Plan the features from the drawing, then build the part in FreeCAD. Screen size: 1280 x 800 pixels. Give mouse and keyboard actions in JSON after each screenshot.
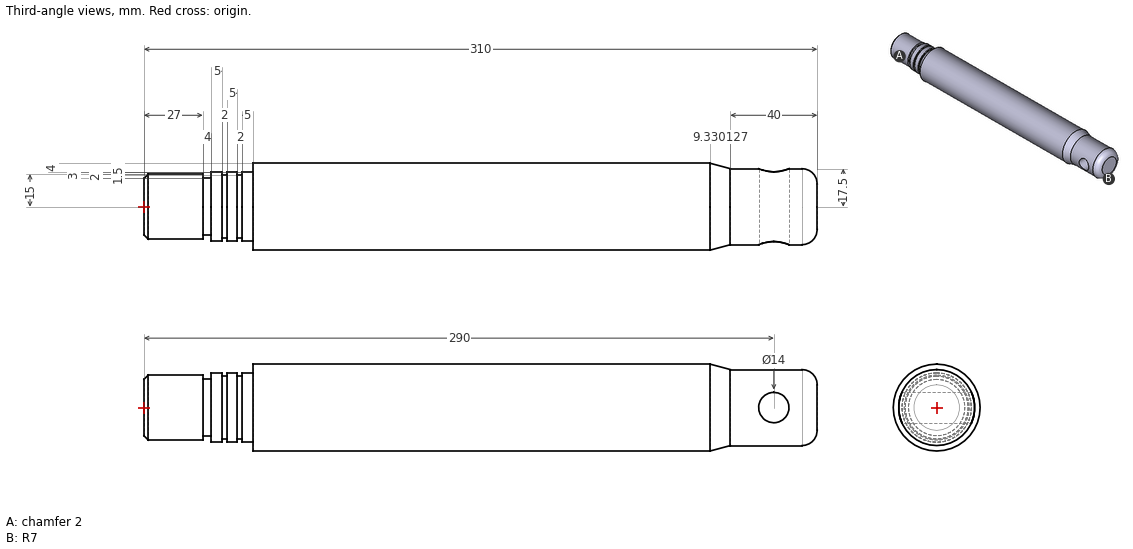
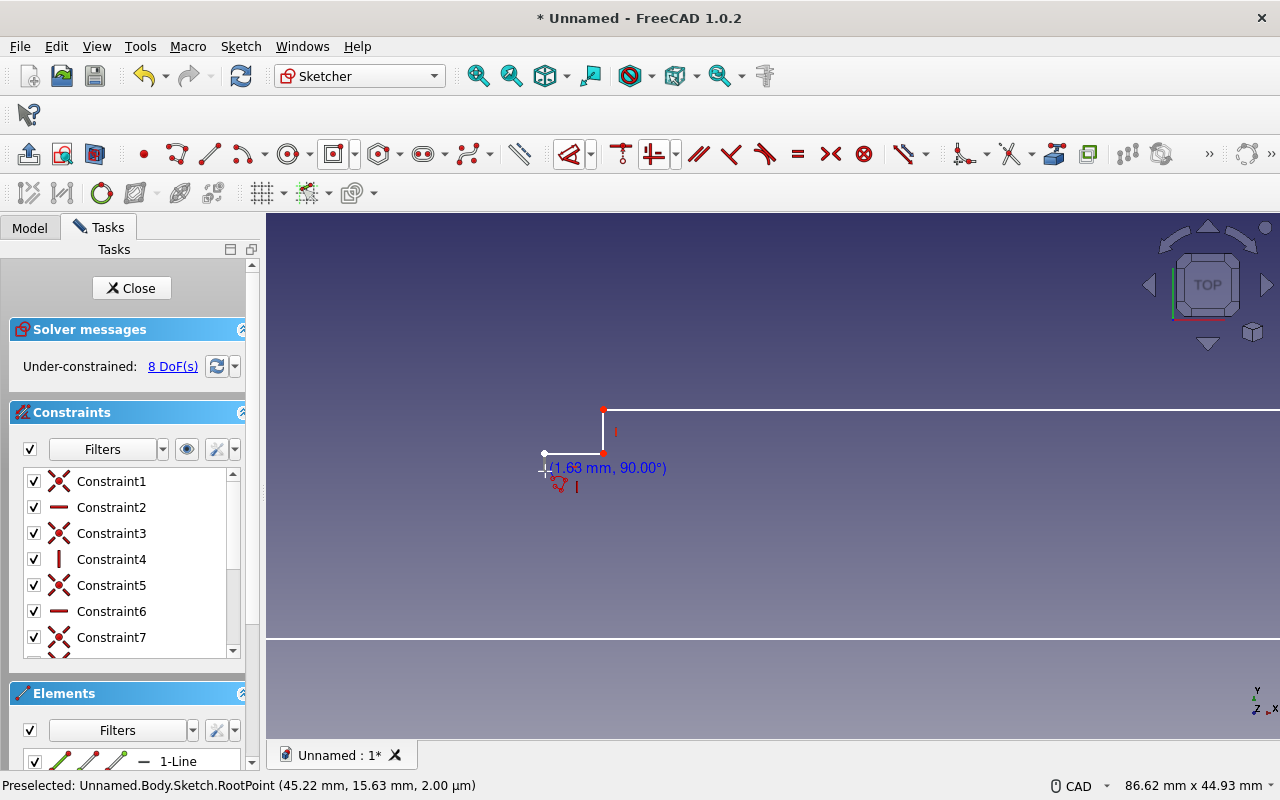
{"action": "left_click", "coordinate": [545, 470]}
{"action": "left_click", "coordinate": [521, 470]}
{"action": "left_click", "coordinate": [521, 452]}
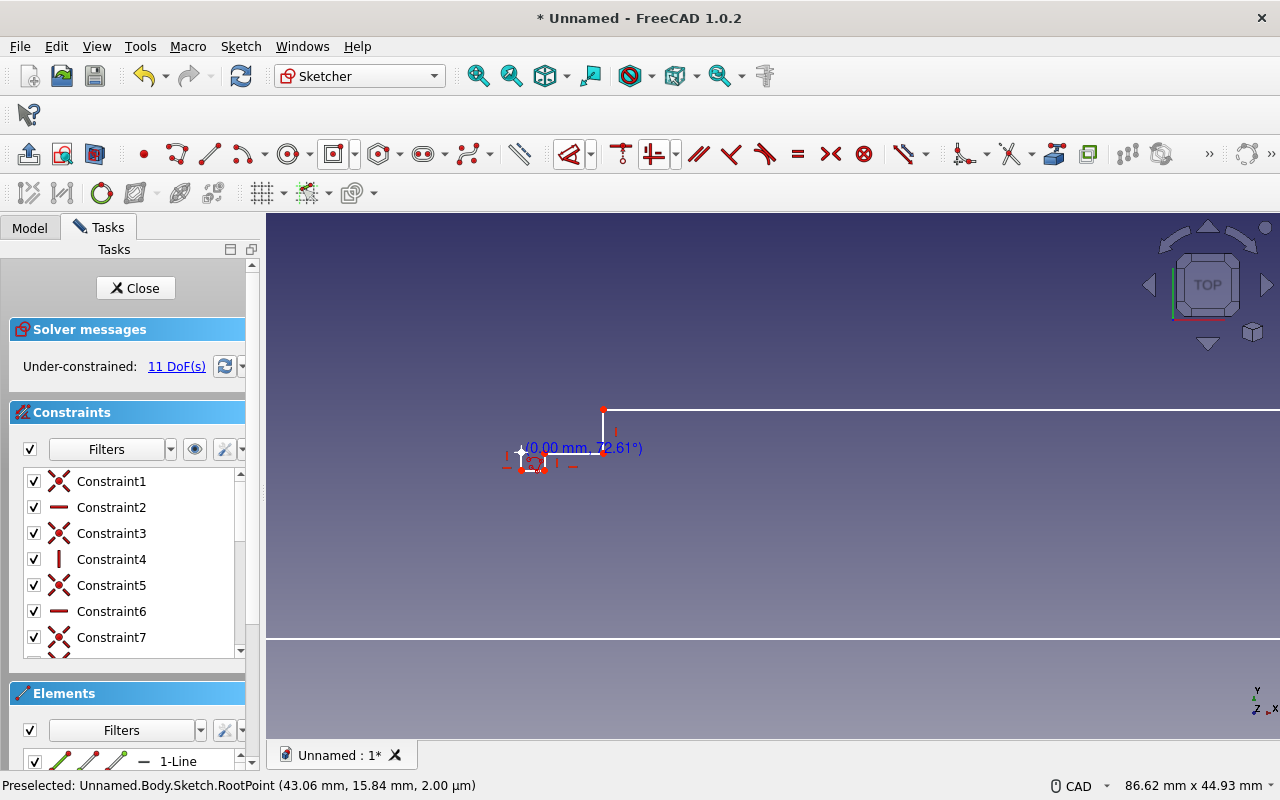
{"action": "scroll", "coordinate": [481, 467], "scroll_direction": "down", "scroll_amount": 9}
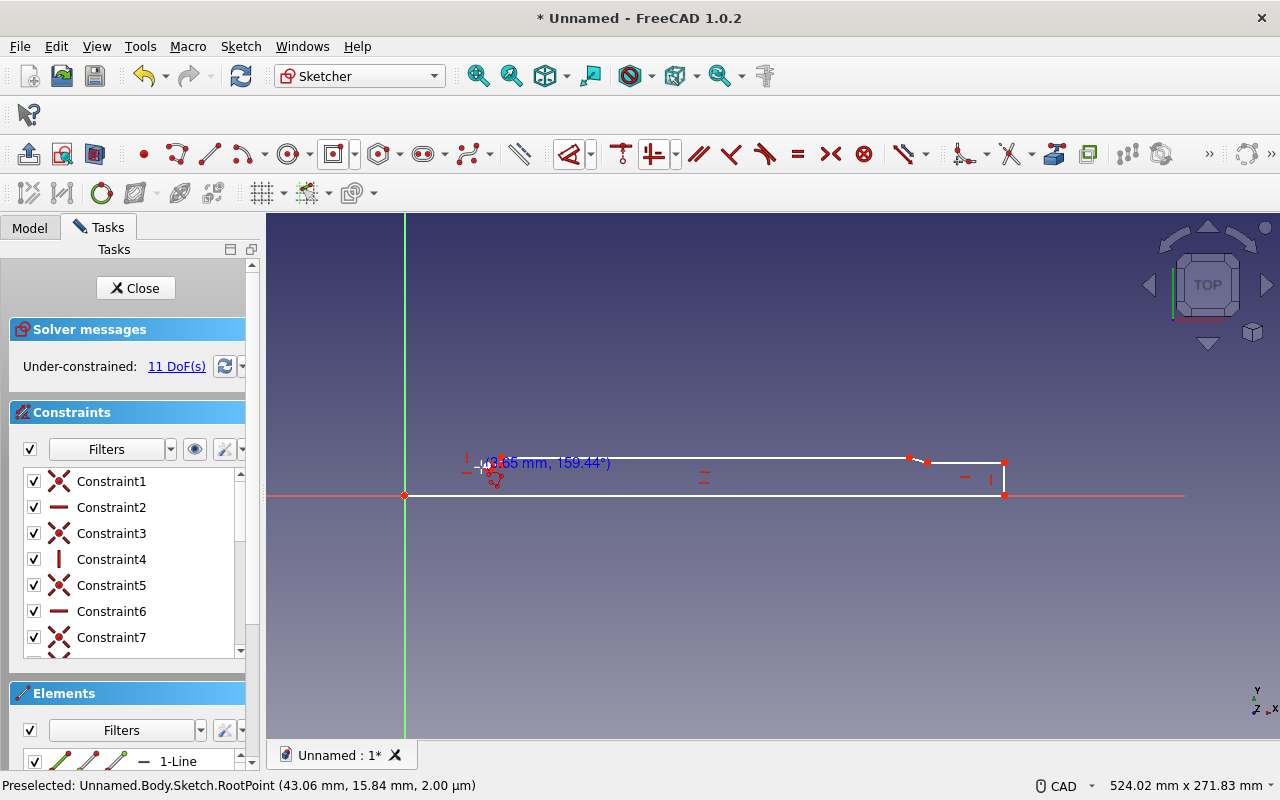
{"action": "scroll", "coordinate": [478, 465], "scroll_direction": "up", "scroll_amount": 3}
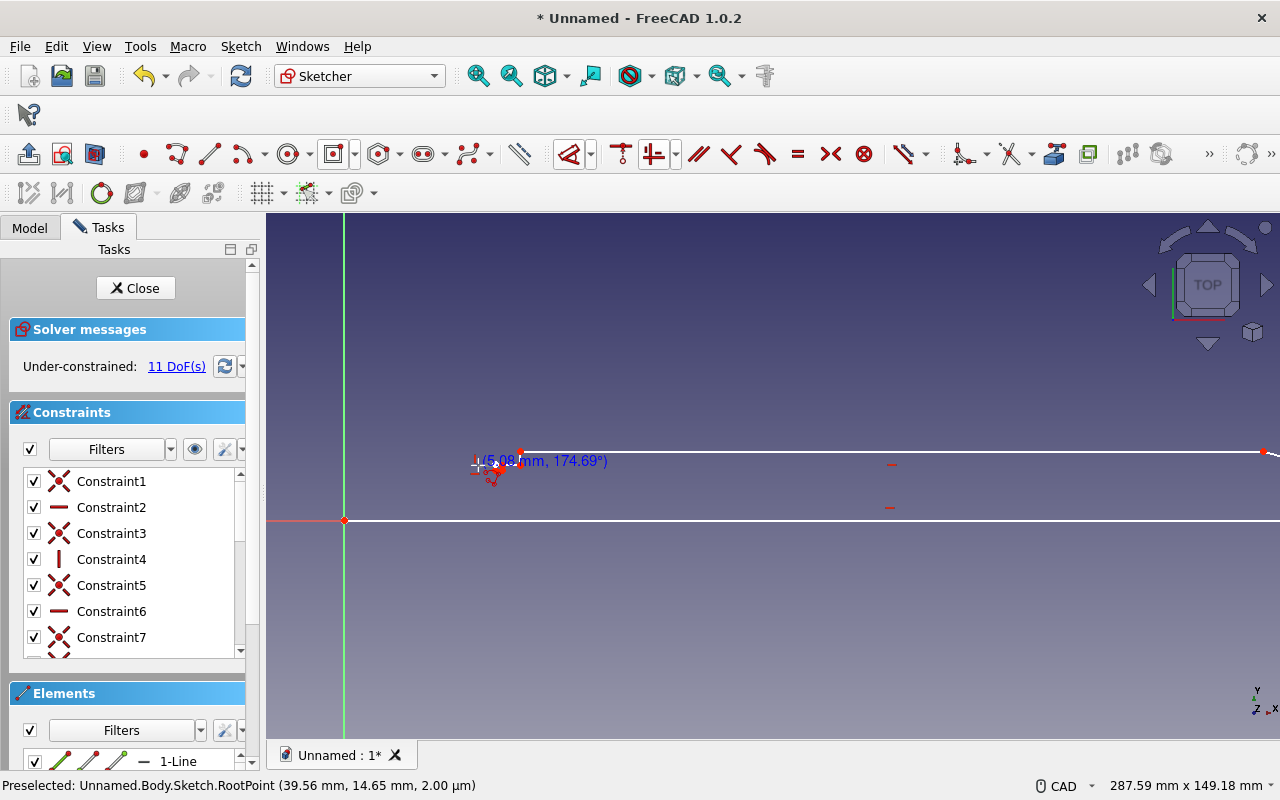
{"action": "left_click", "coordinate": [478, 464]}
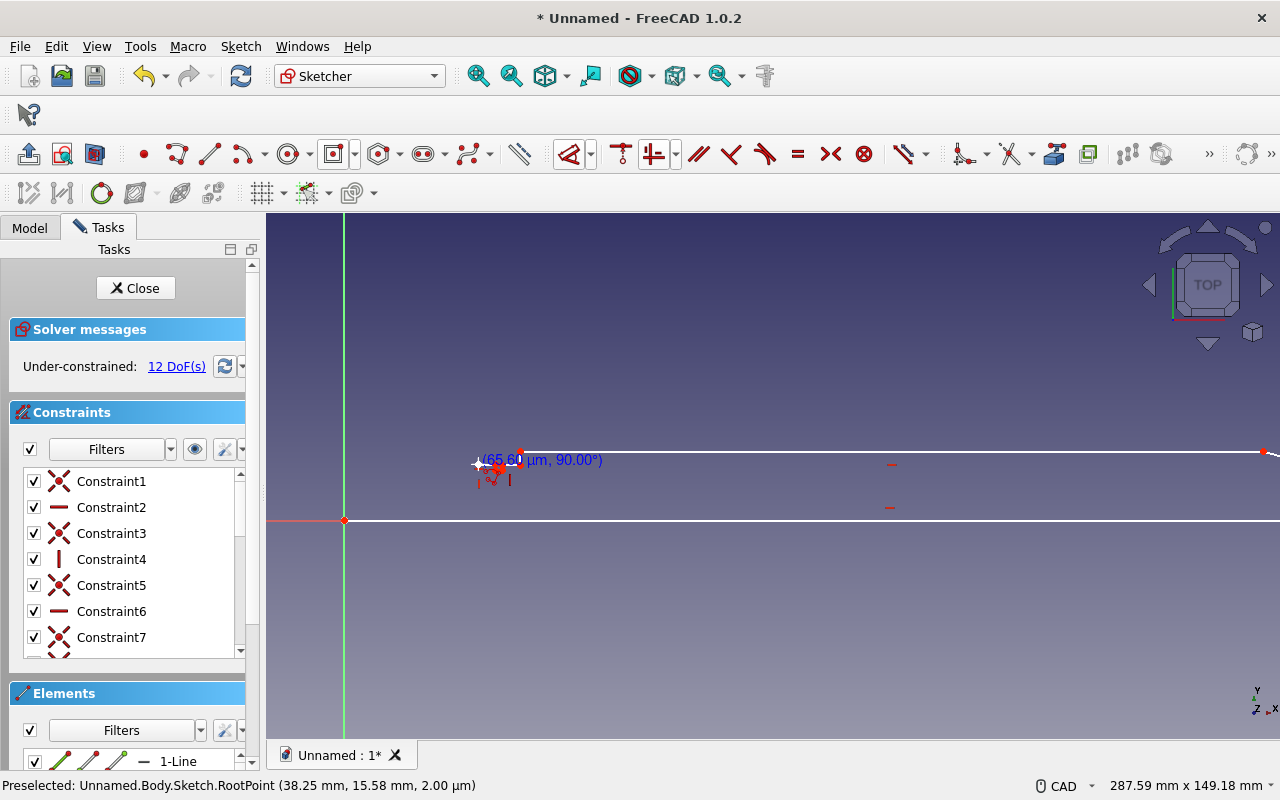
{"action": "scroll", "coordinate": [478, 470], "scroll_direction": "up", "scroll_amount": 6}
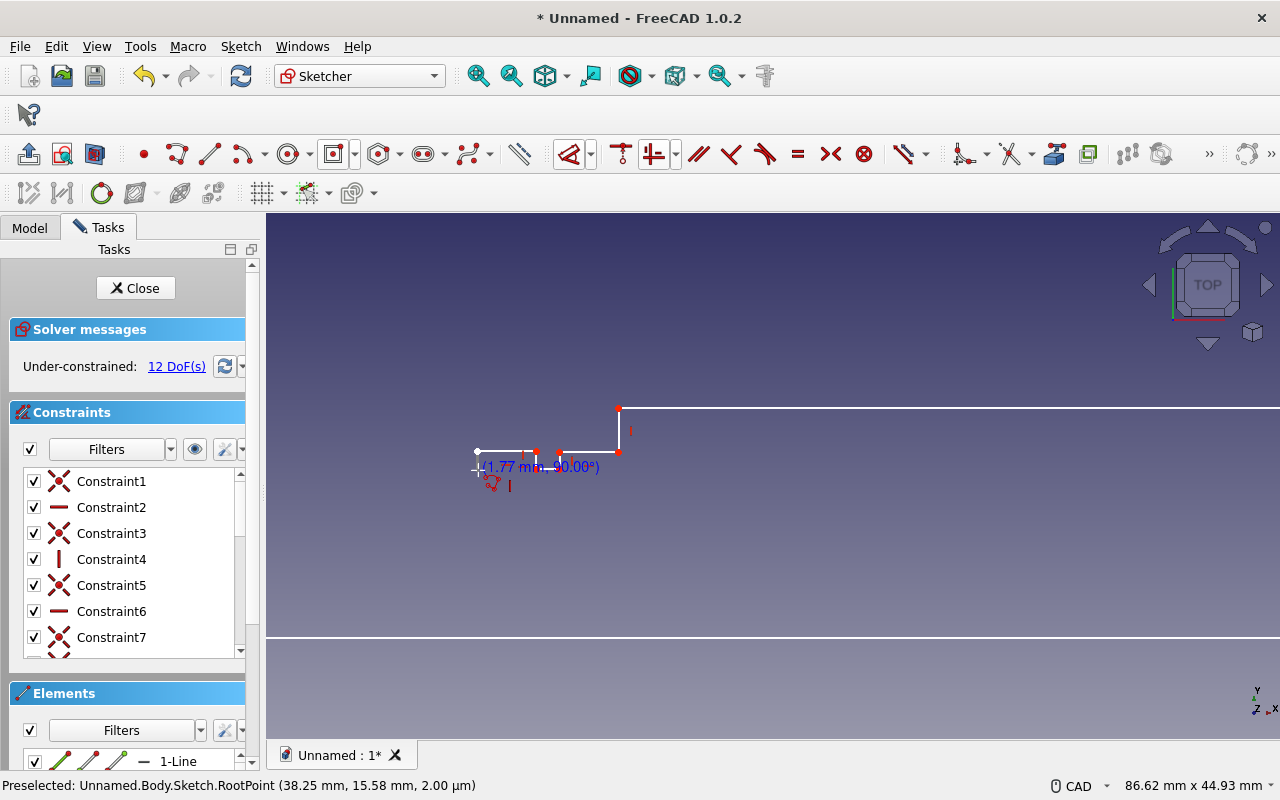
{"action": "left_click", "coordinate": [478, 468]}
{"action": "left_click", "coordinate": [455, 468]}
{"action": "left_click", "coordinate": [455, 451]}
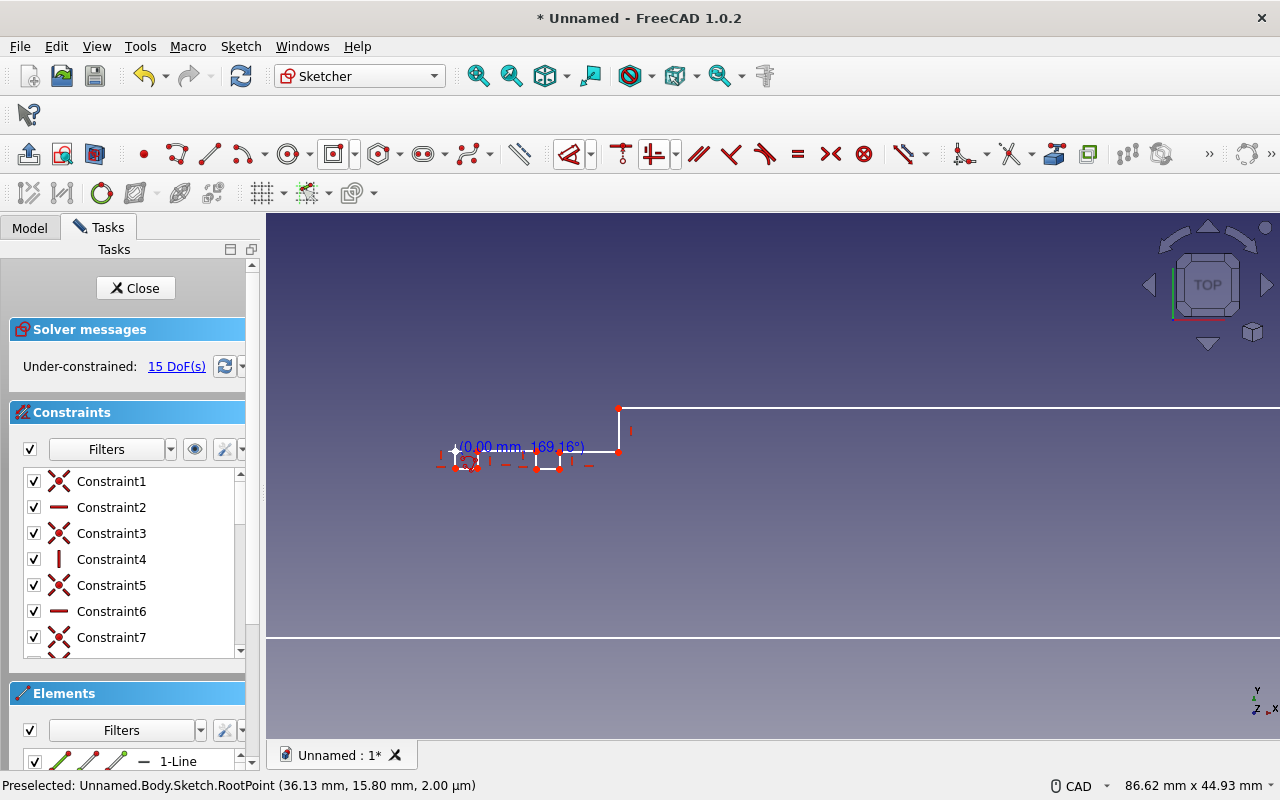
{"action": "scroll", "coordinate": [478, 467], "scroll_direction": "down", "scroll_amount": 9}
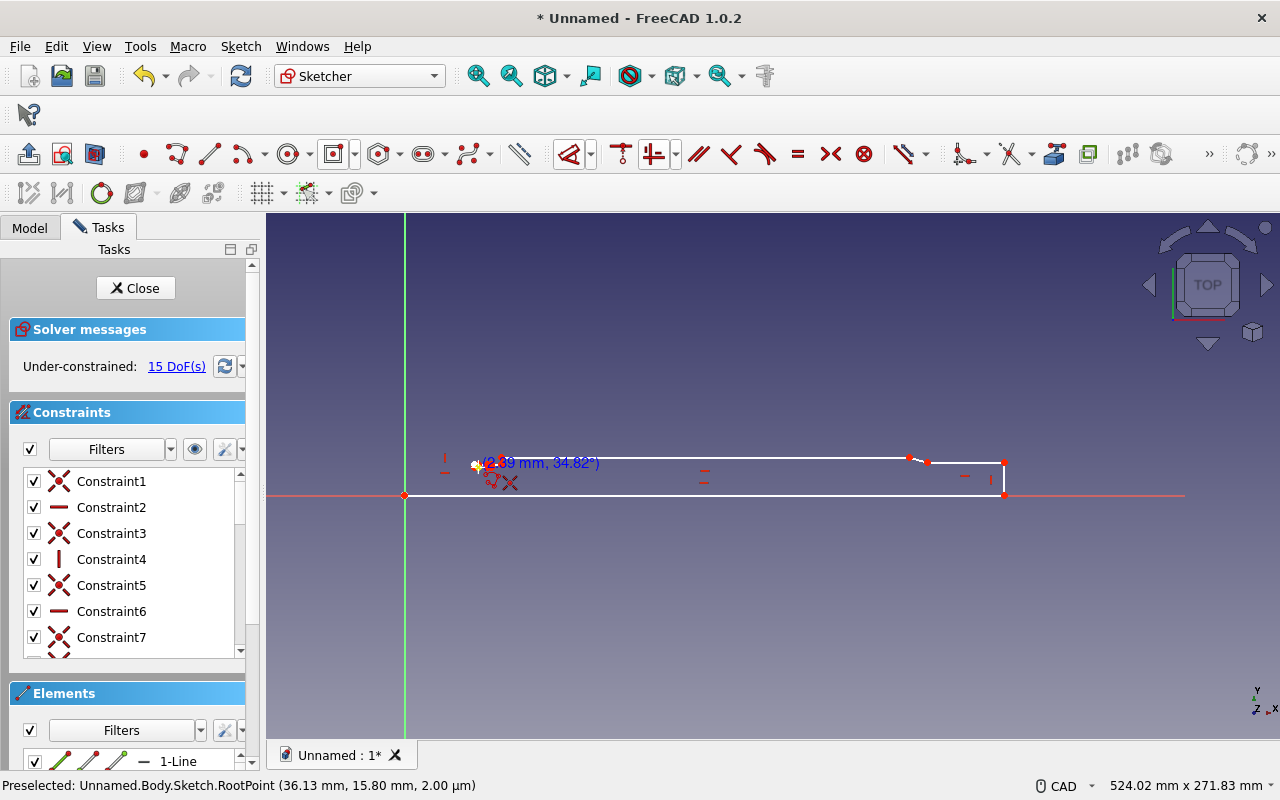
{"action": "scroll", "coordinate": [465, 465], "scroll_direction": "up", "scroll_amount": 3}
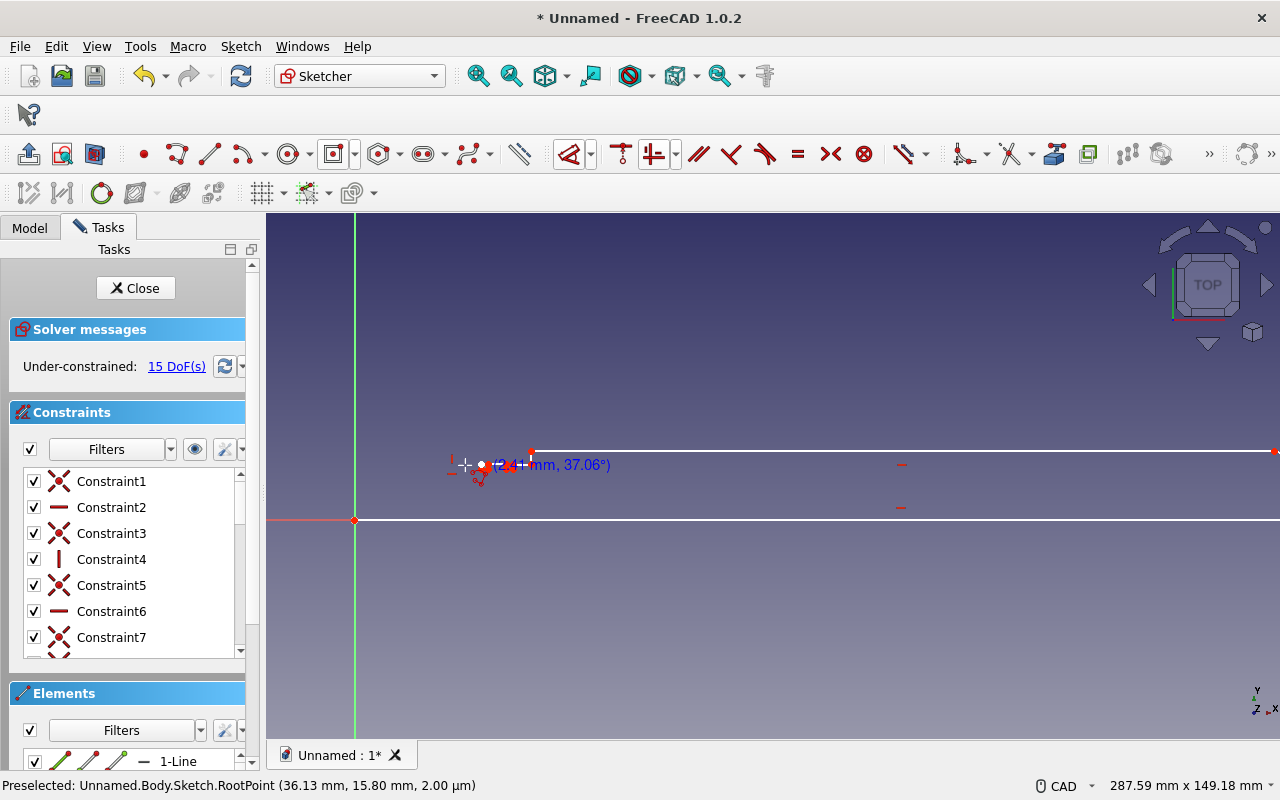
{"action": "left_click", "coordinate": [464, 464]}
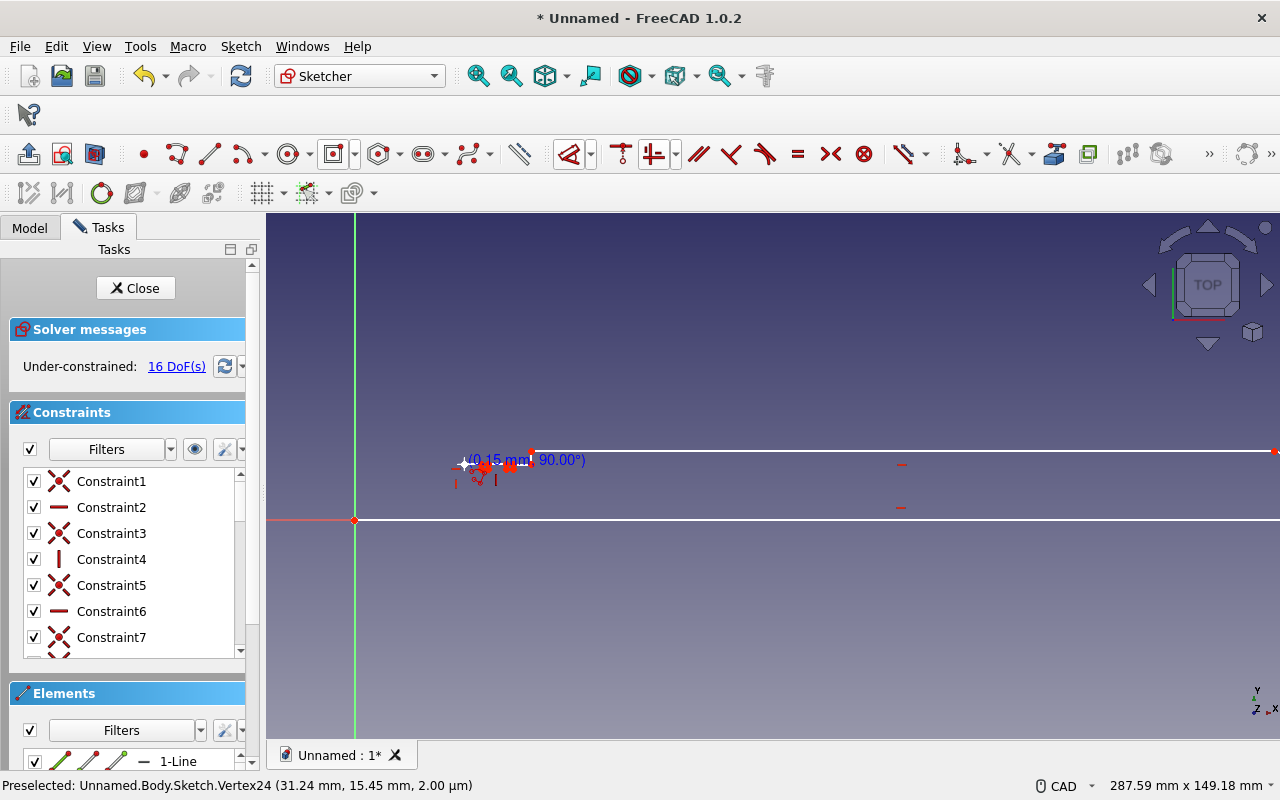
{"action": "scroll", "coordinate": [464, 475], "scroll_direction": "up", "scroll_amount": 3}